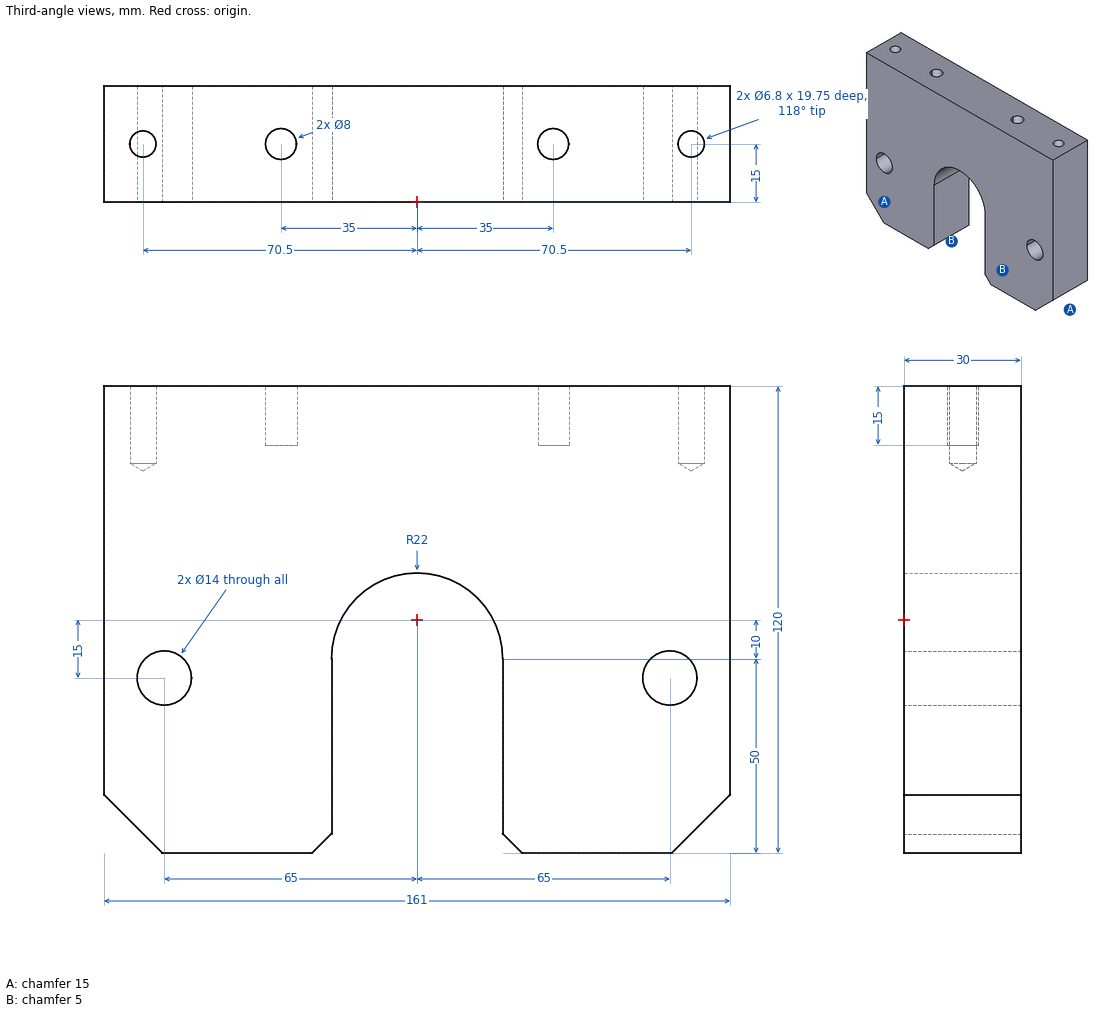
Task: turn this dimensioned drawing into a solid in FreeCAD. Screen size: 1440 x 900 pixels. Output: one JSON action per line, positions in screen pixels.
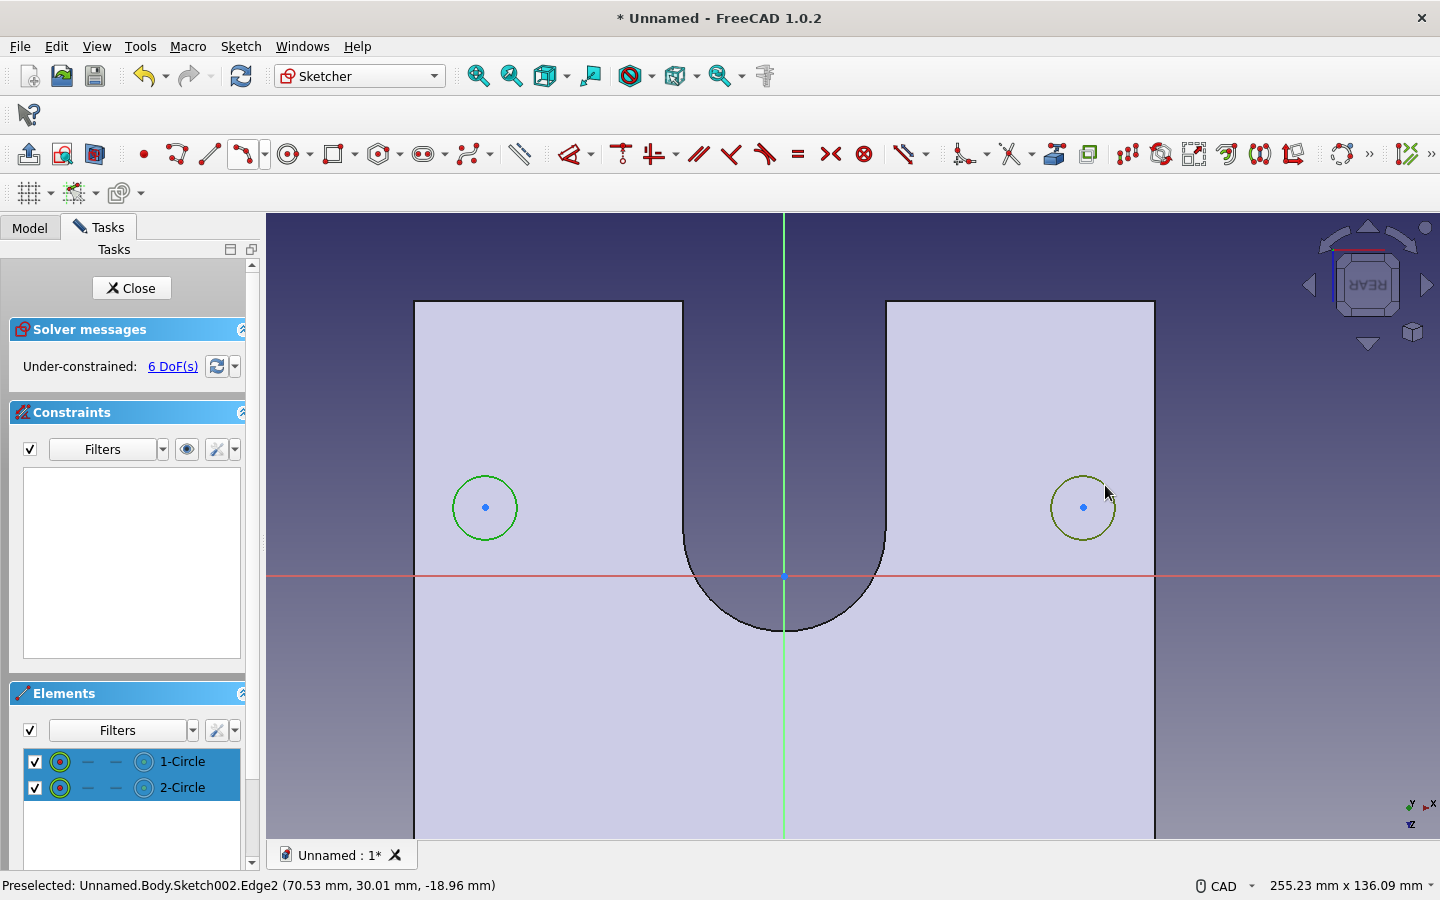
{"action": "left_click", "coordinate": [798, 154]}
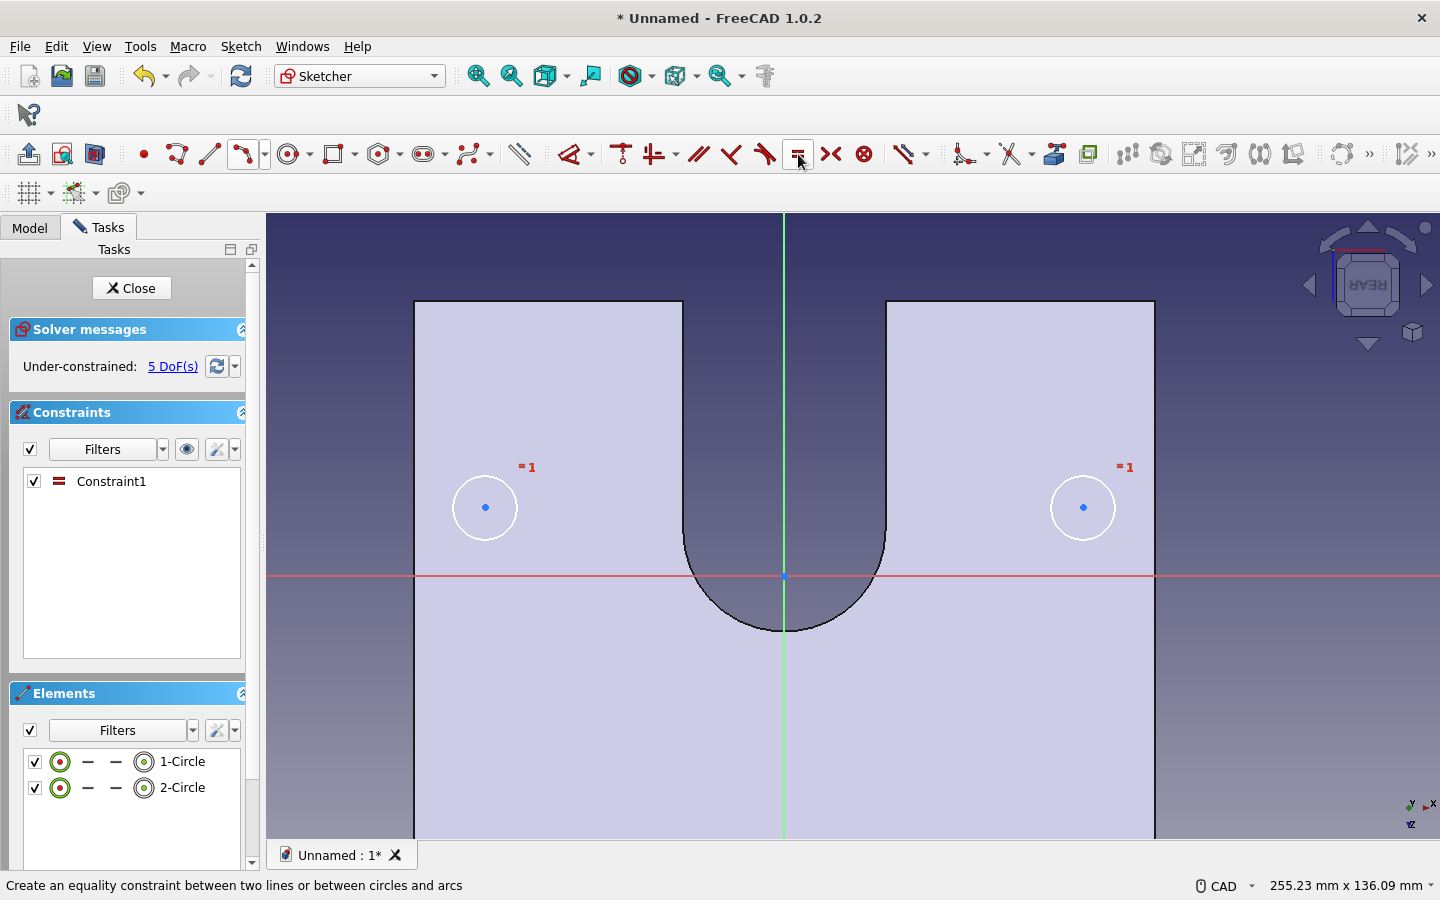
{"action": "left_click", "coordinate": [485, 508]}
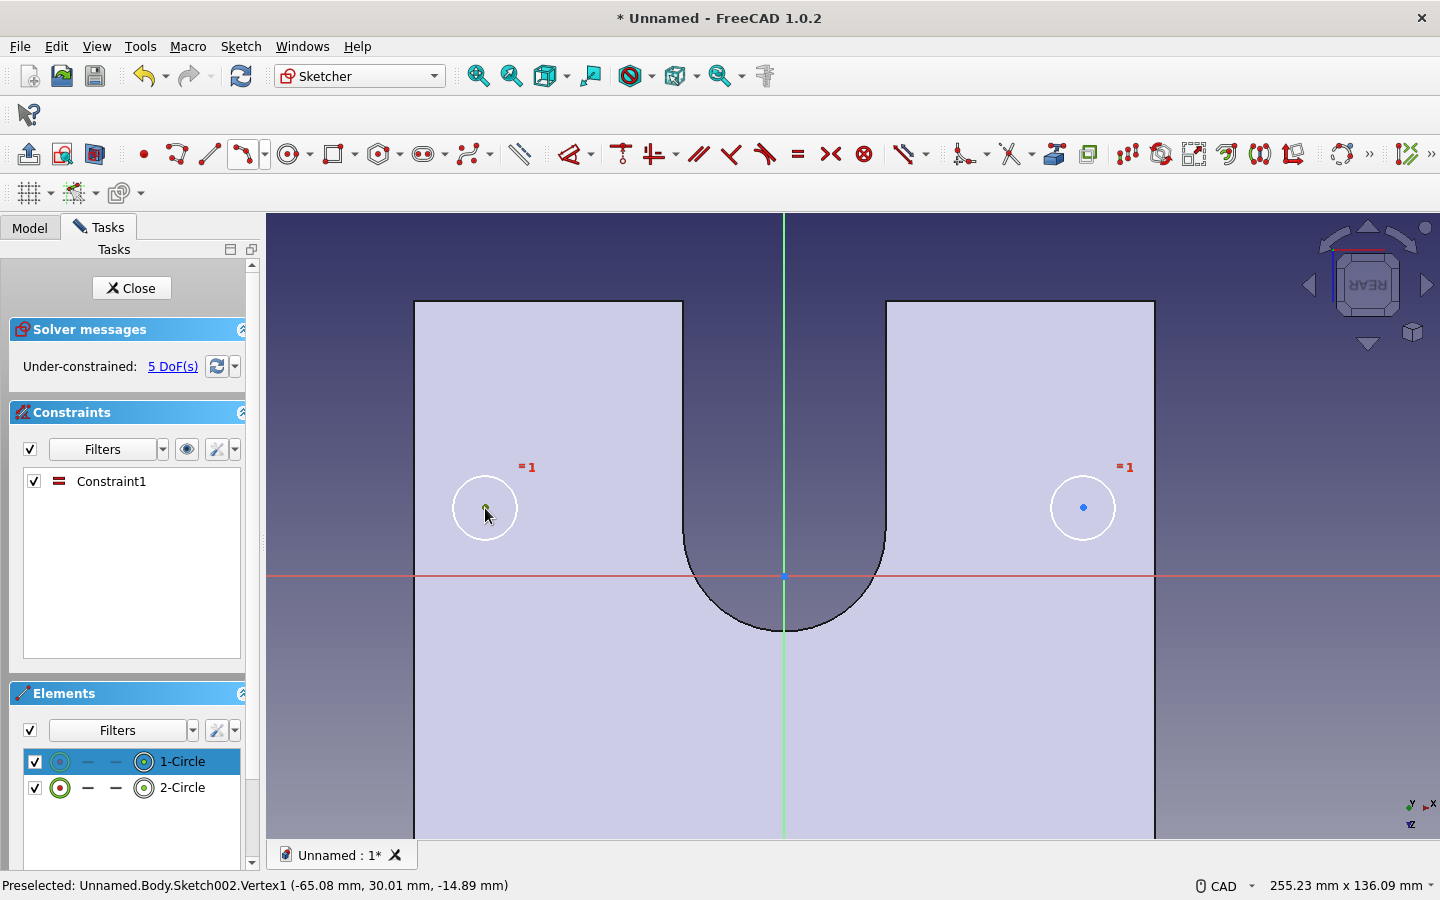
{"action": "left_click", "coordinate": [1083, 508]}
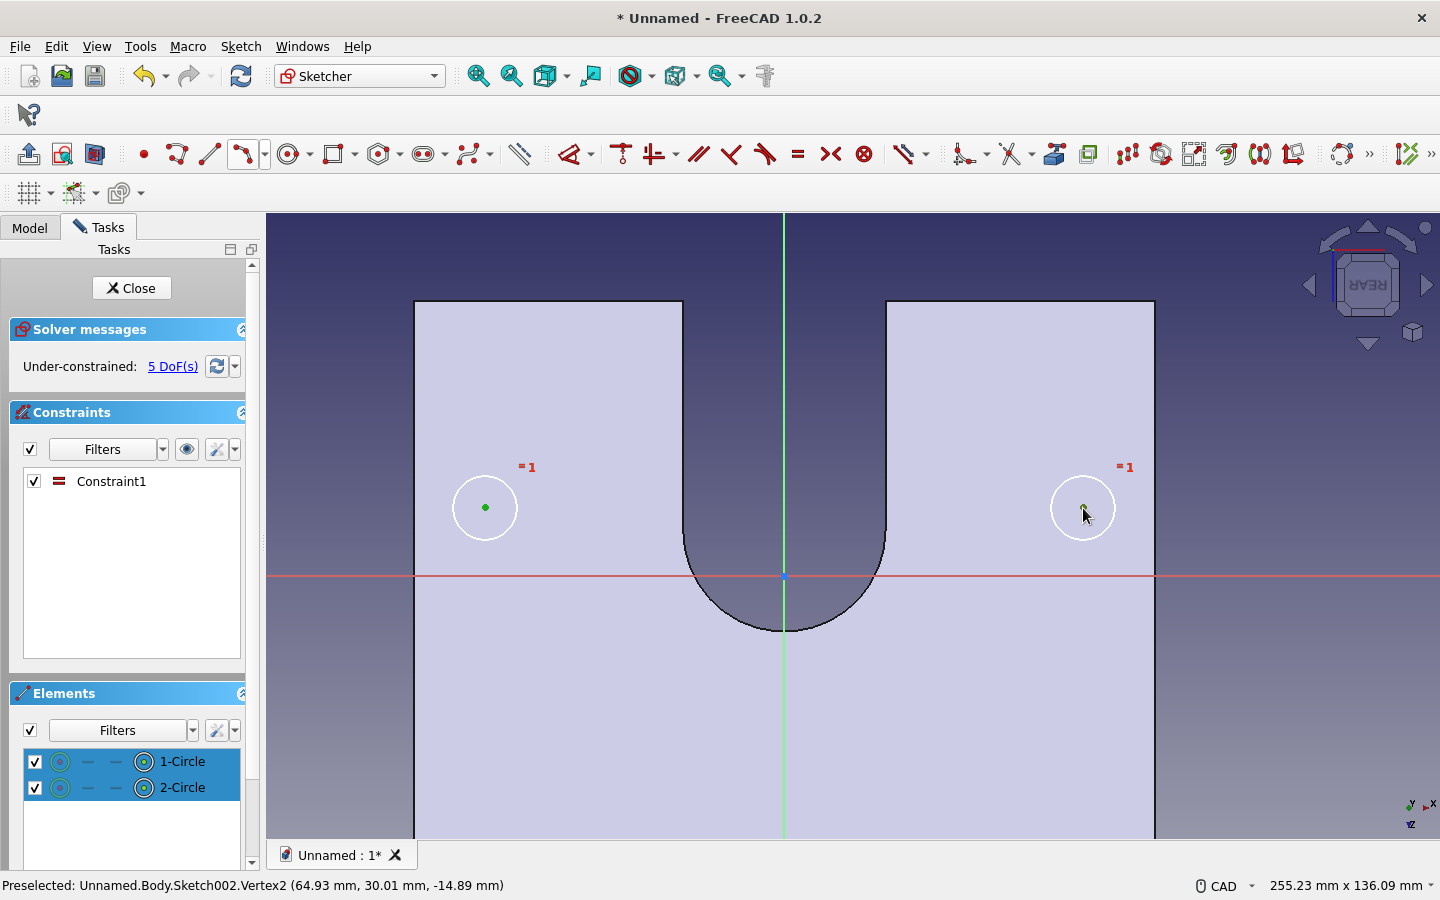
{"action": "key", "text": "h"}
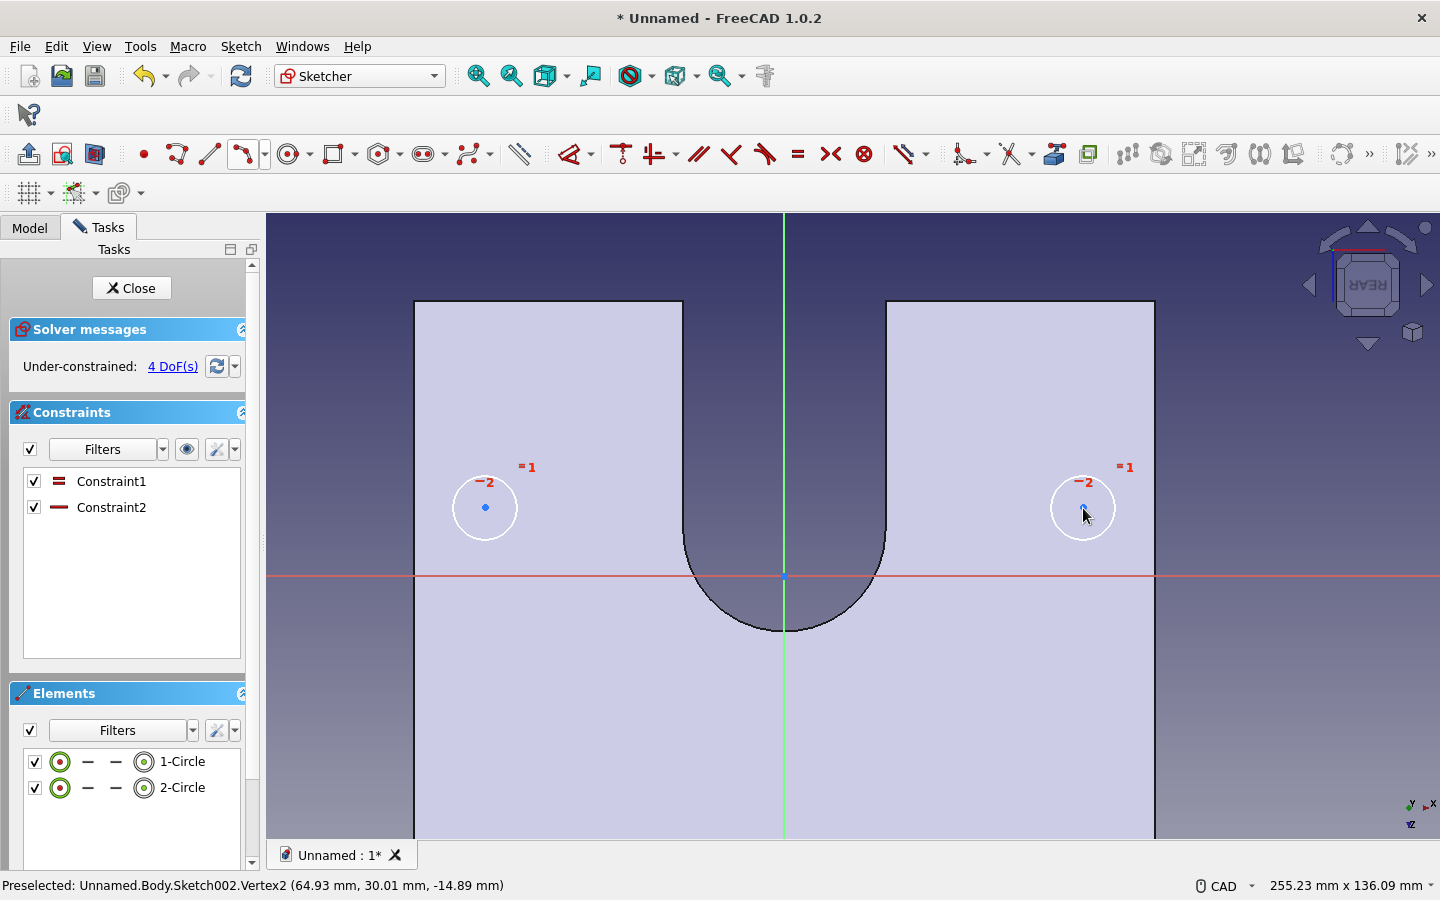
{"action": "key", "text": "d"}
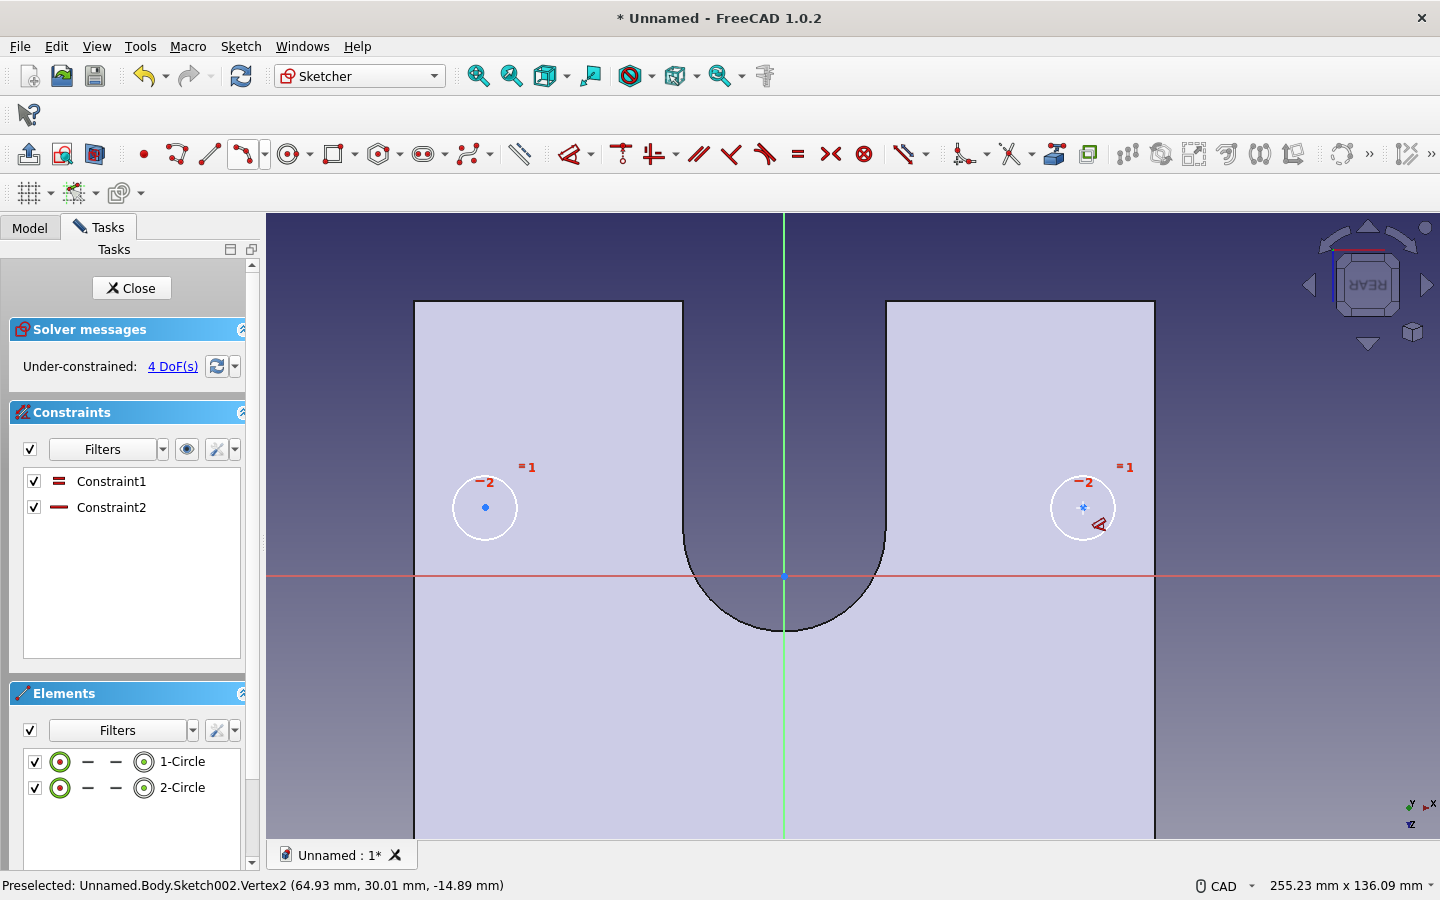
{"action": "left_click", "coordinate": [507, 485]}
{"action": "left_click", "coordinate": [529, 462]}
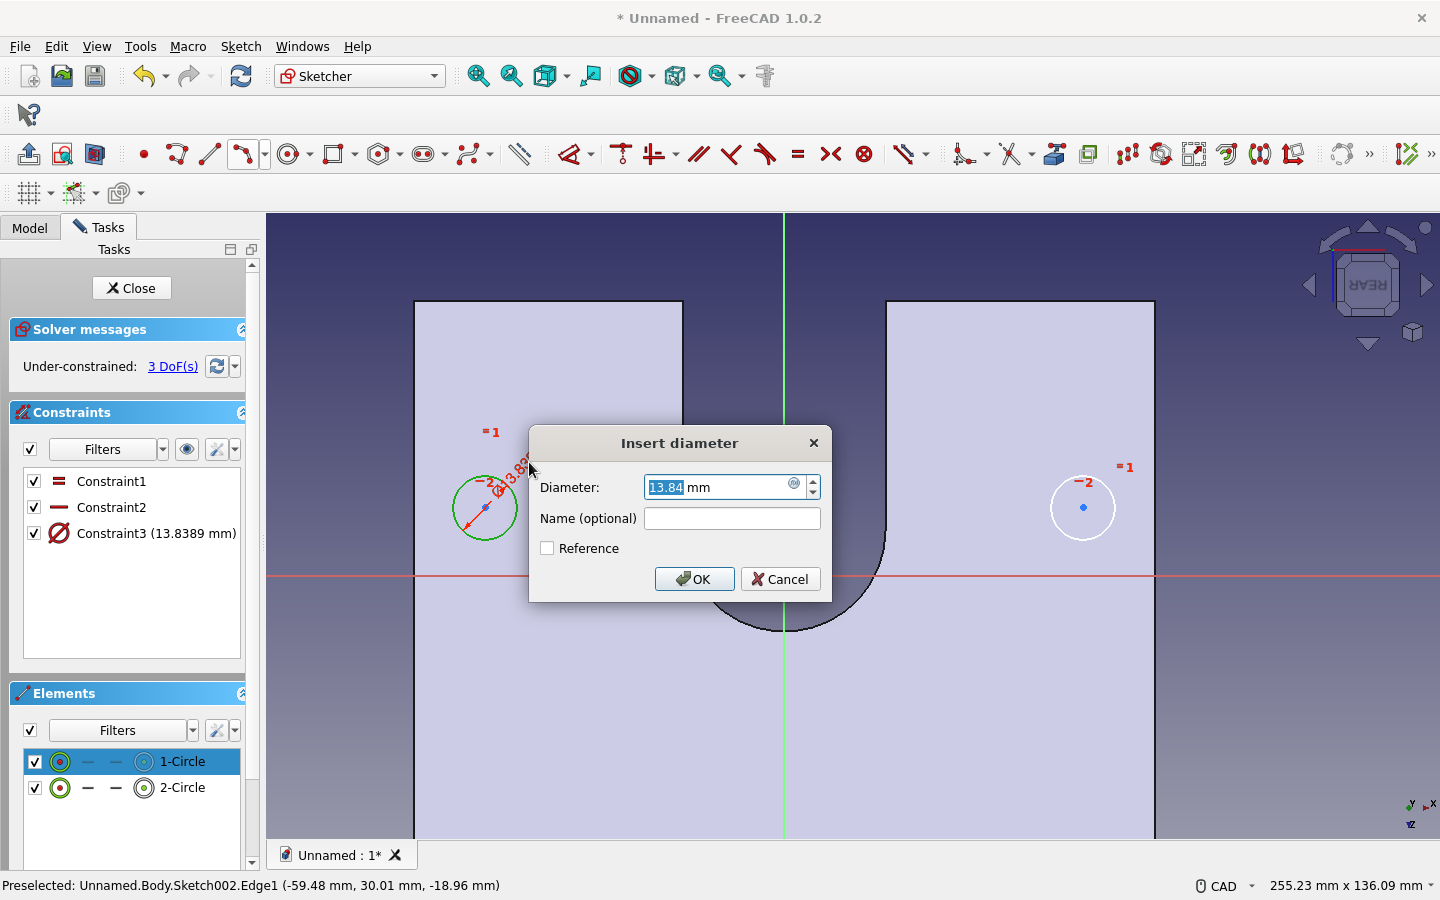
{"action": "type", "text": "14"}
{"action": "key", "text": "Return"}